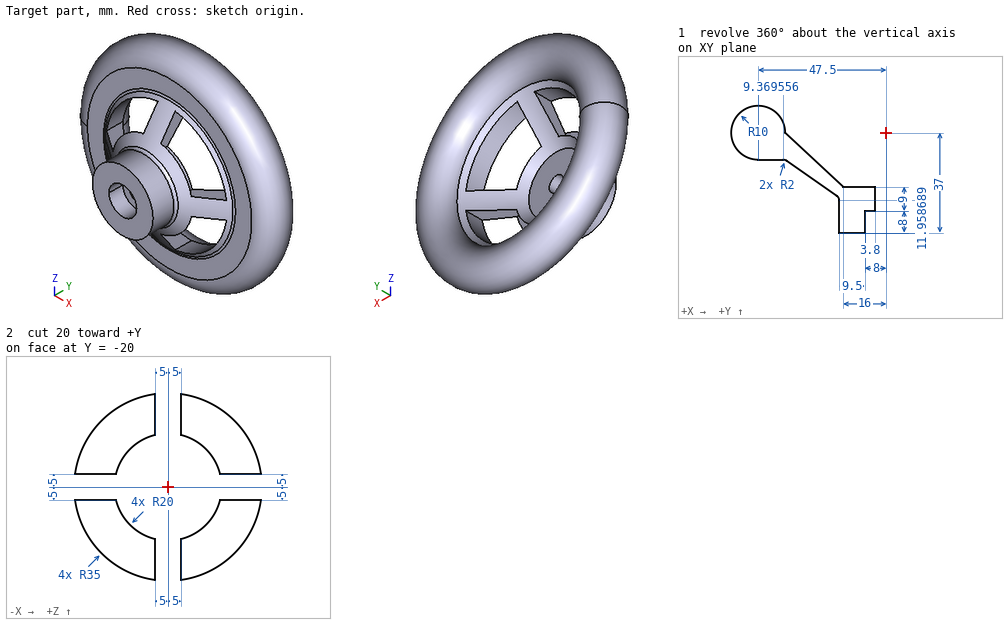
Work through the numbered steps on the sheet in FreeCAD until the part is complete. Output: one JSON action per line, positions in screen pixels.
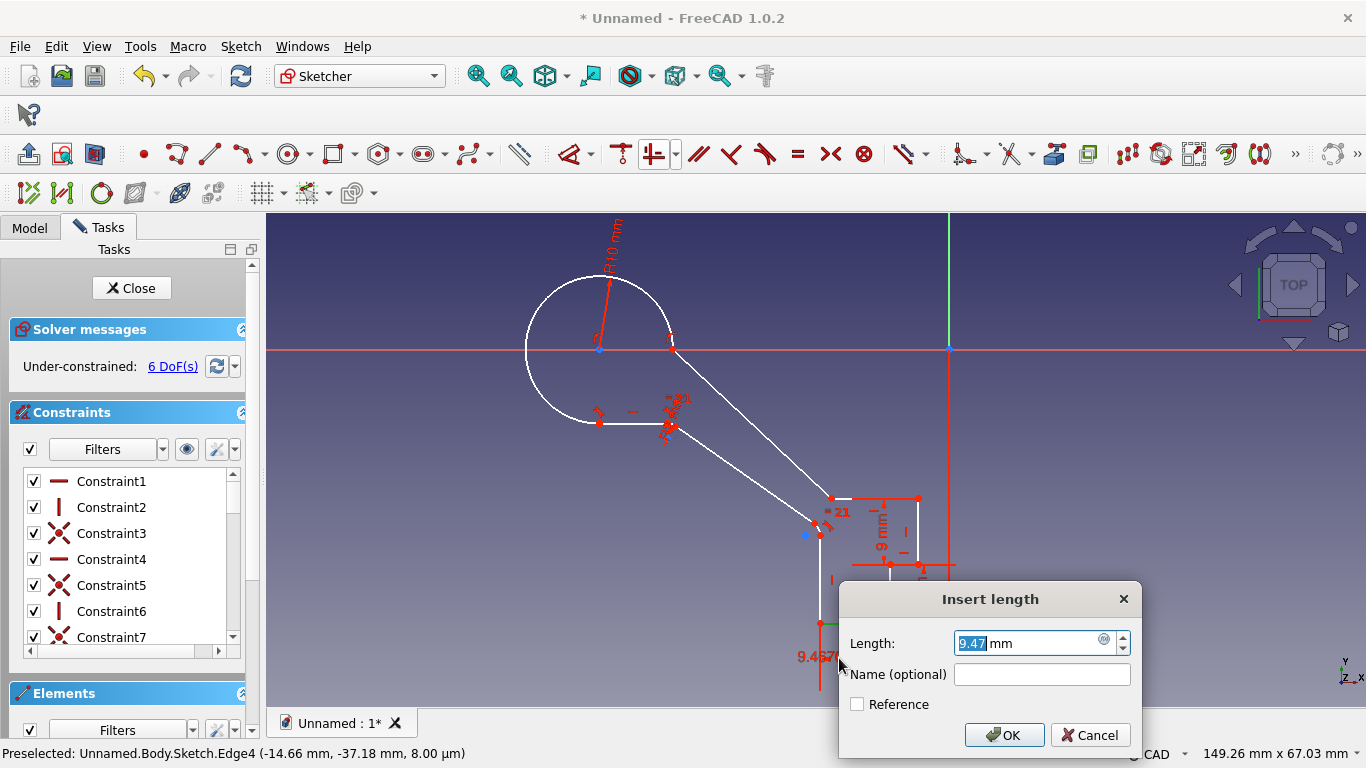
{"action": "type", "text": "9.5"}
{"action": "key", "text": "Return"}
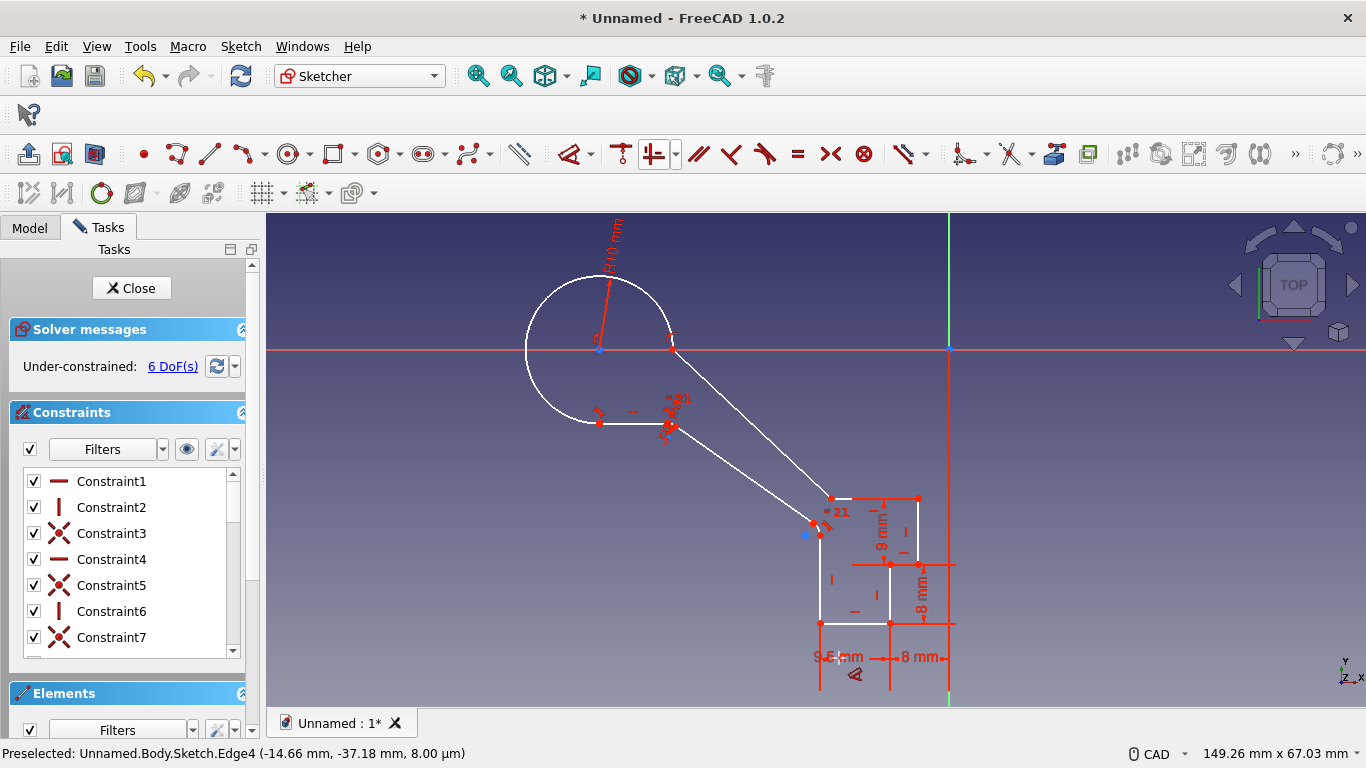
{"action": "scroll", "coordinate": [901, 565], "scroll_direction": "up", "scroll_amount": 2}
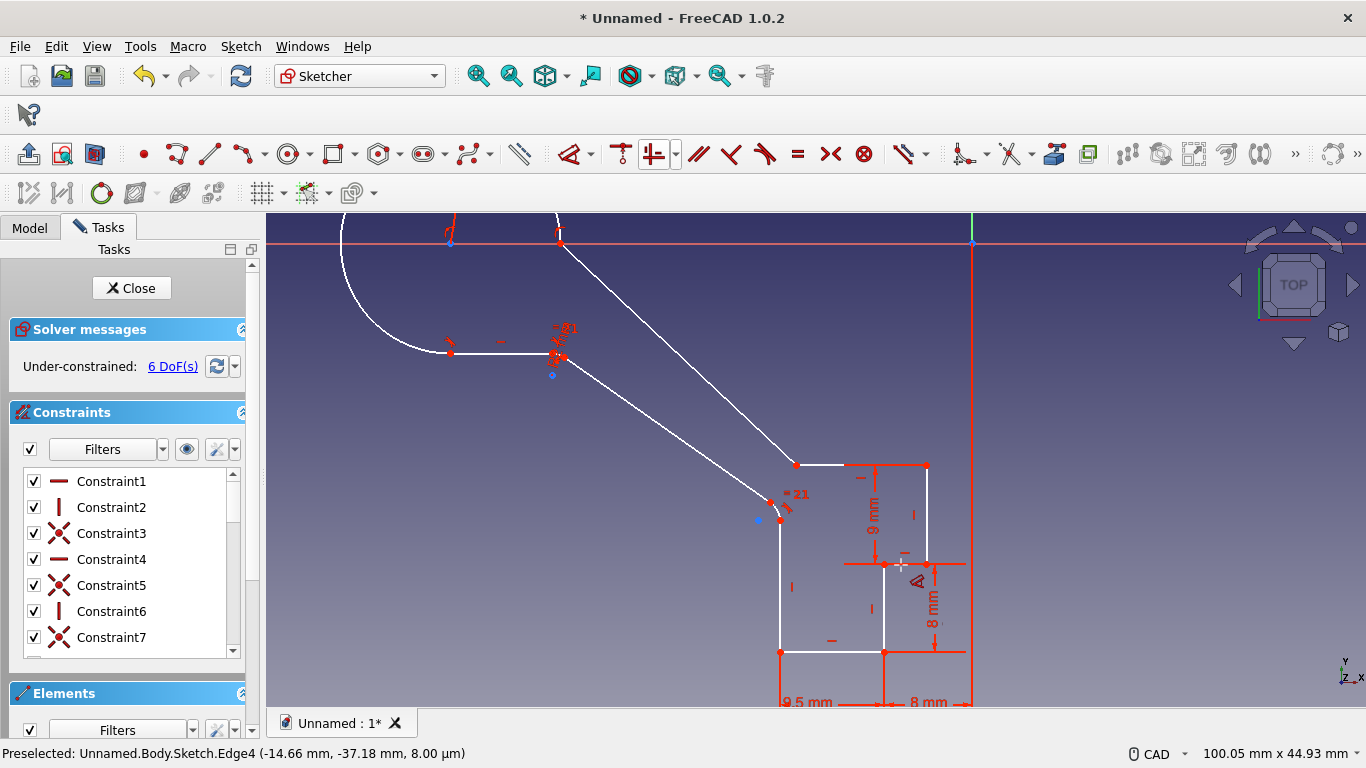
{"action": "left_click", "coordinate": [901, 564]}
{"action": "left_click", "coordinate": [906, 646]}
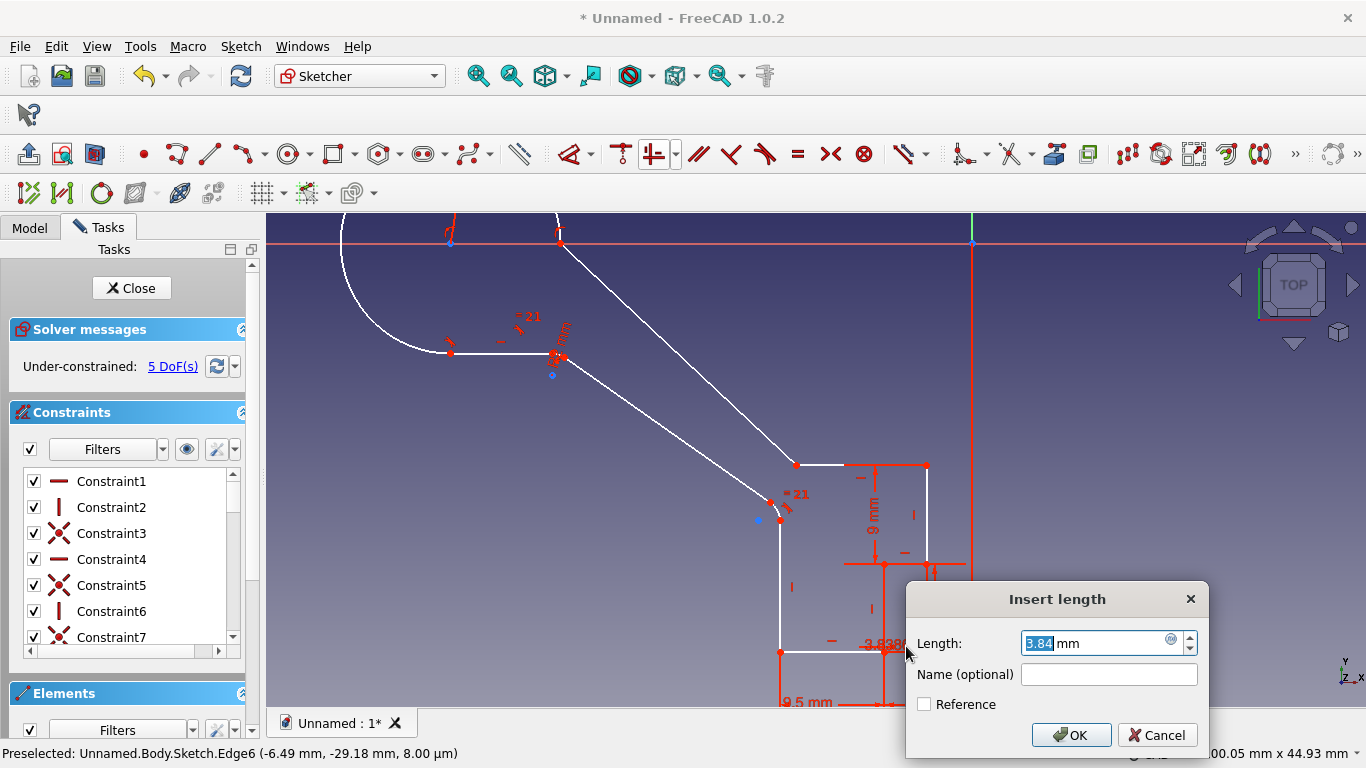
{"action": "type", "text": "3.8"}
{"action": "key", "text": "Return"}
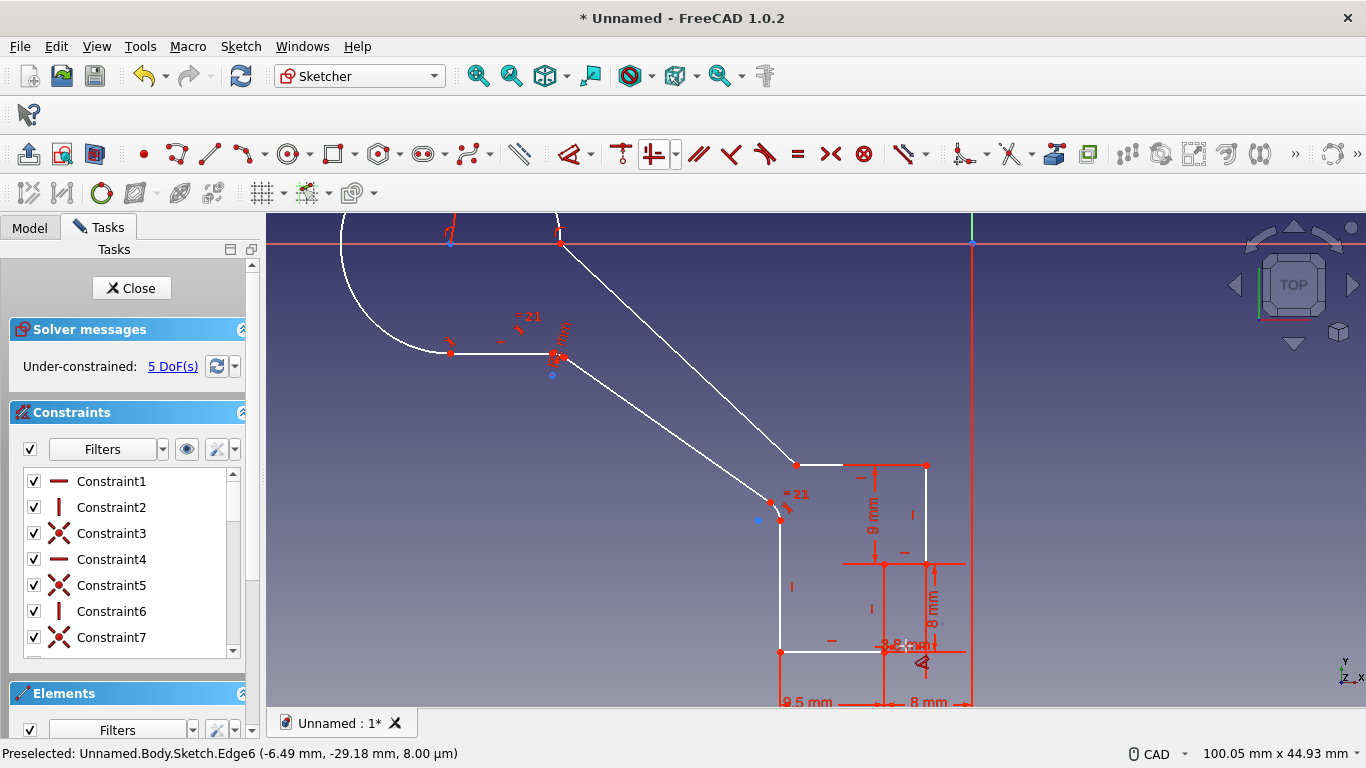
{"action": "left_click", "coordinate": [780, 652]}
{"action": "left_click", "coordinate": [1006, 448]}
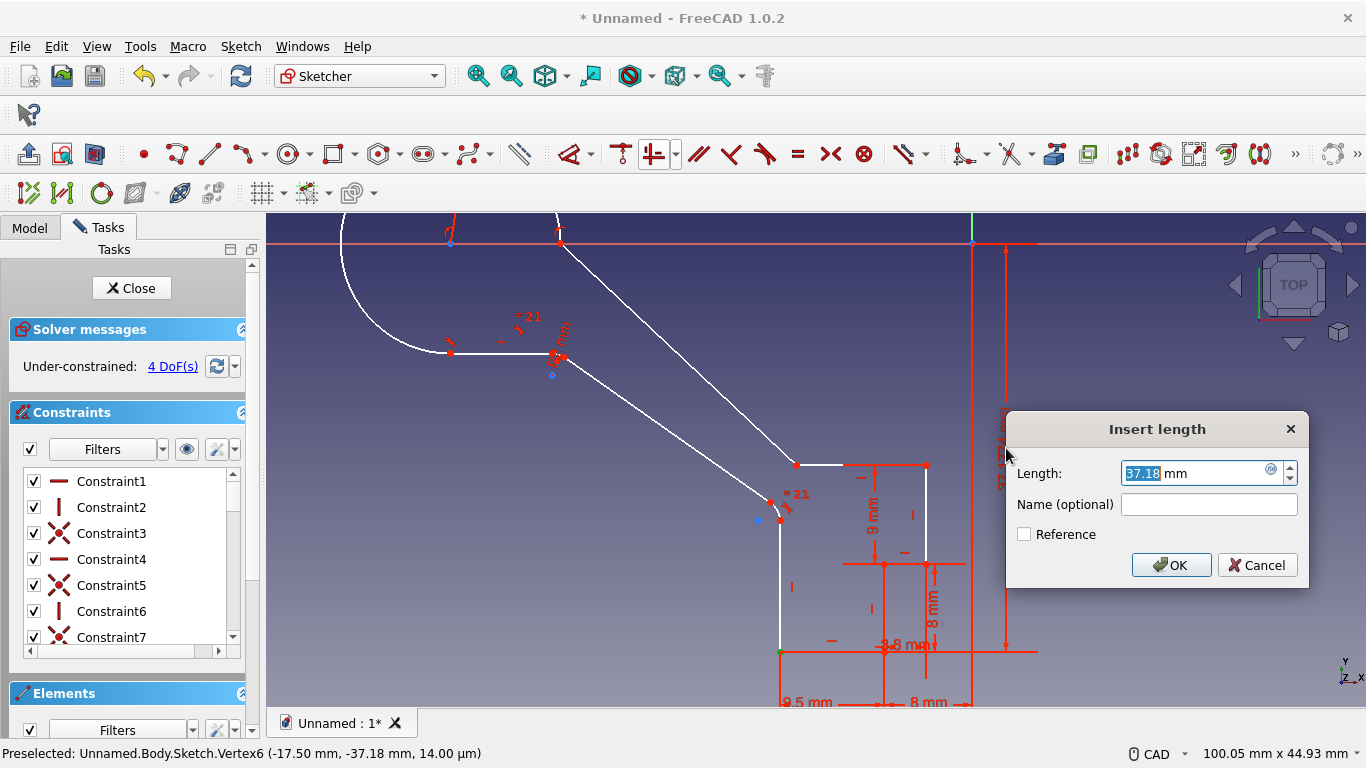
{"action": "type", "text": "37"}
{"action": "key", "text": "Return"}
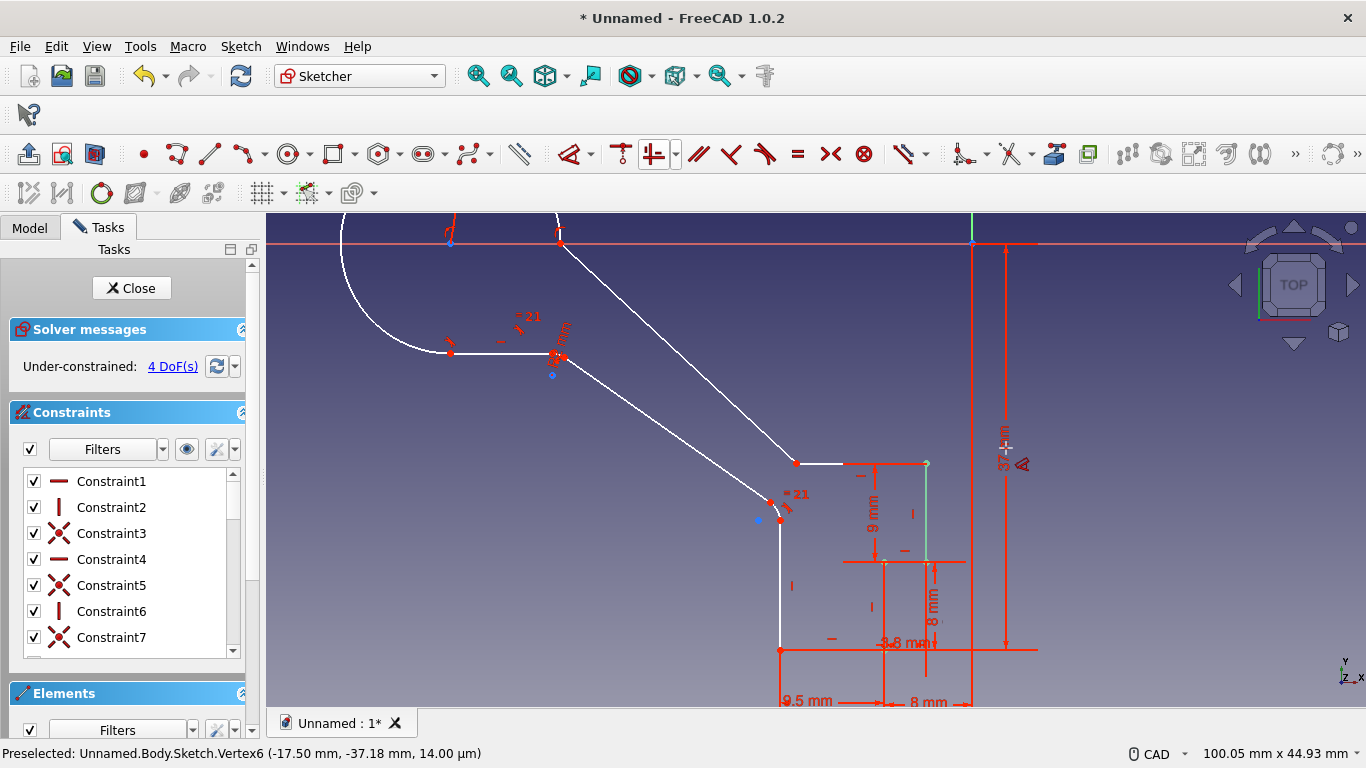
{"action": "left_click", "coordinate": [797, 464]}
{"action": "left_click", "coordinate": [946, 498]}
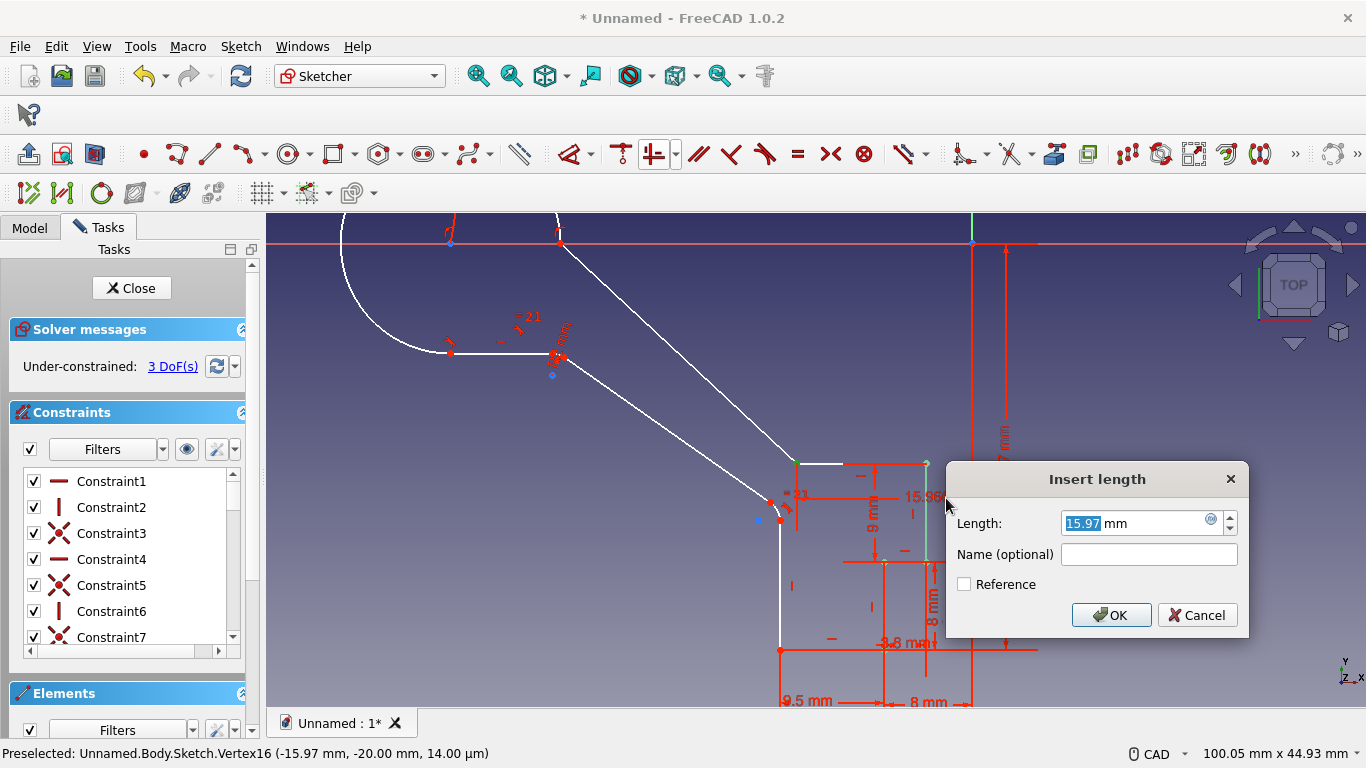
{"action": "type", "text": "16"}
{"action": "key", "text": "Return"}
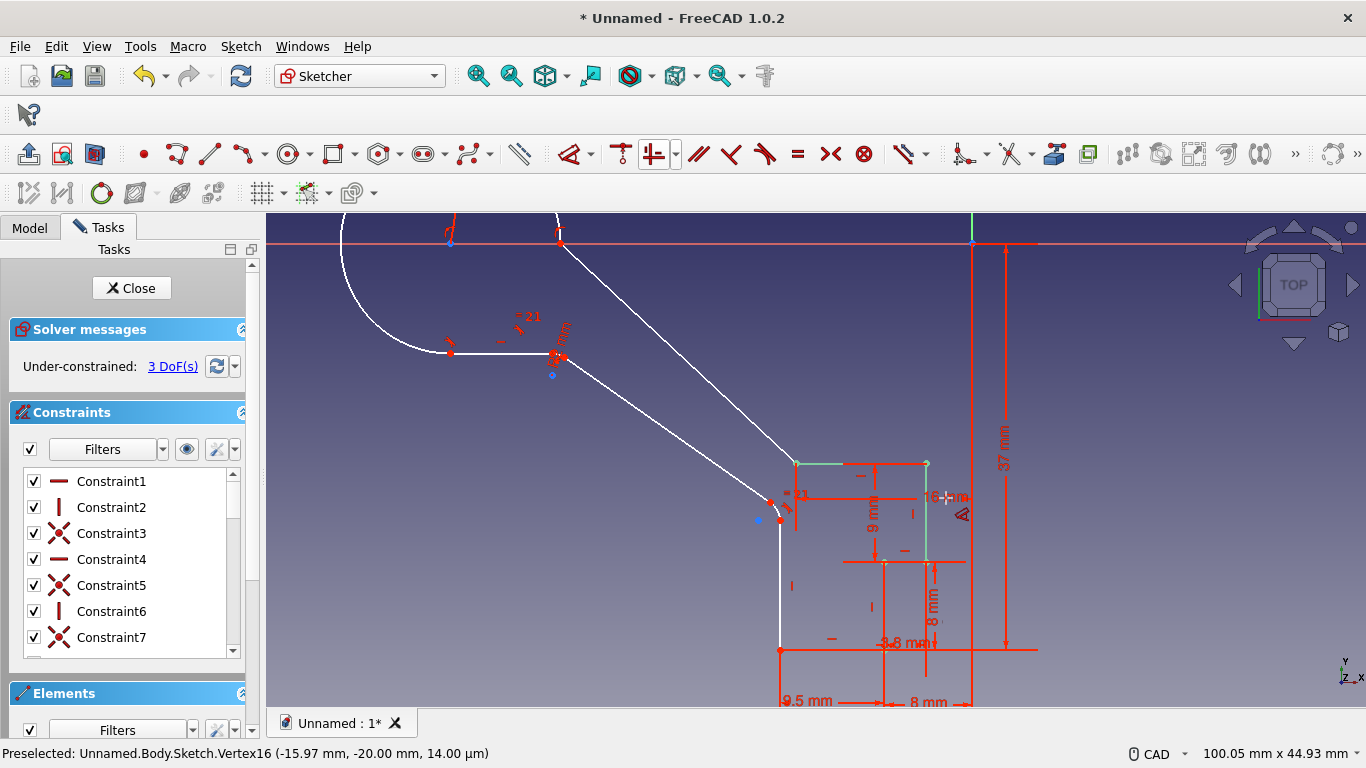
{"action": "left_click", "coordinate": [451, 354]}
{"action": "left_click", "coordinate": [832, 388]}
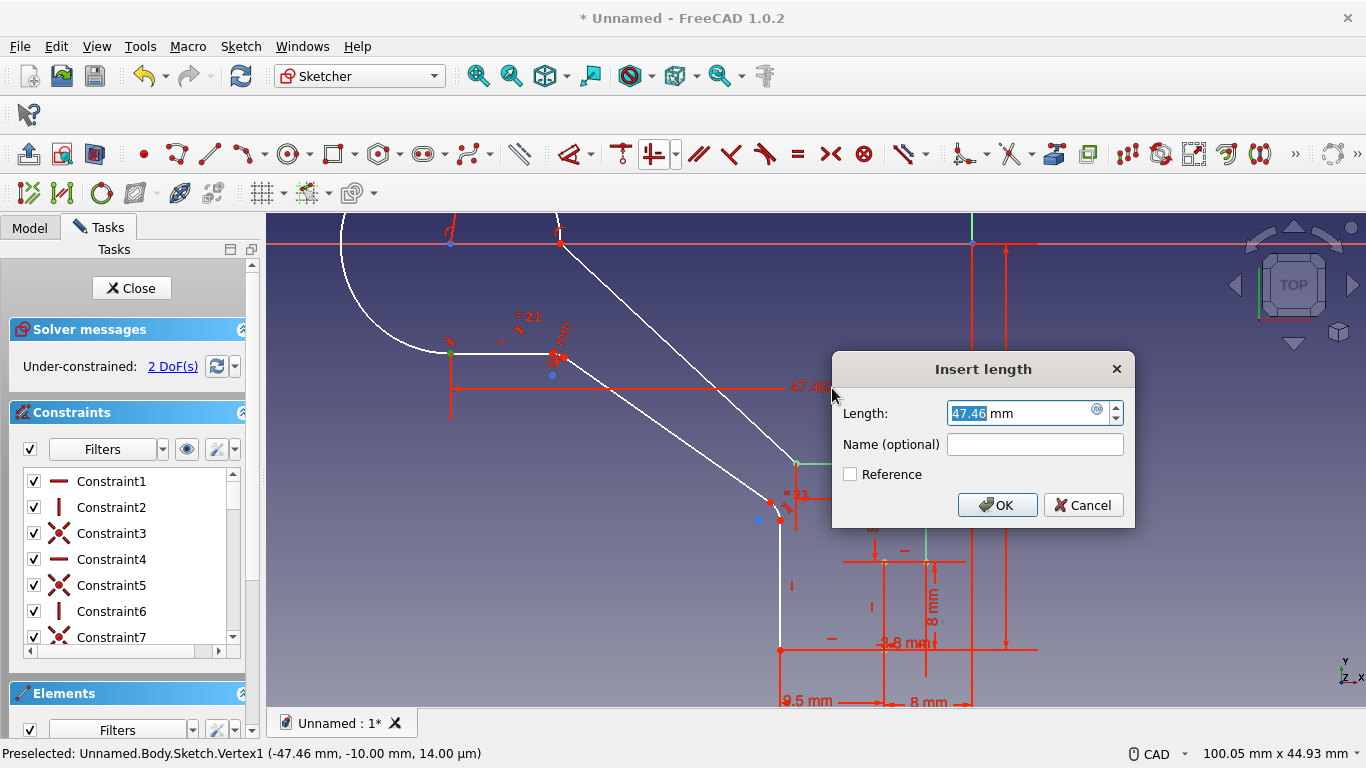
{"action": "type", "text": "47.5"}
{"action": "key", "text": "Return"}